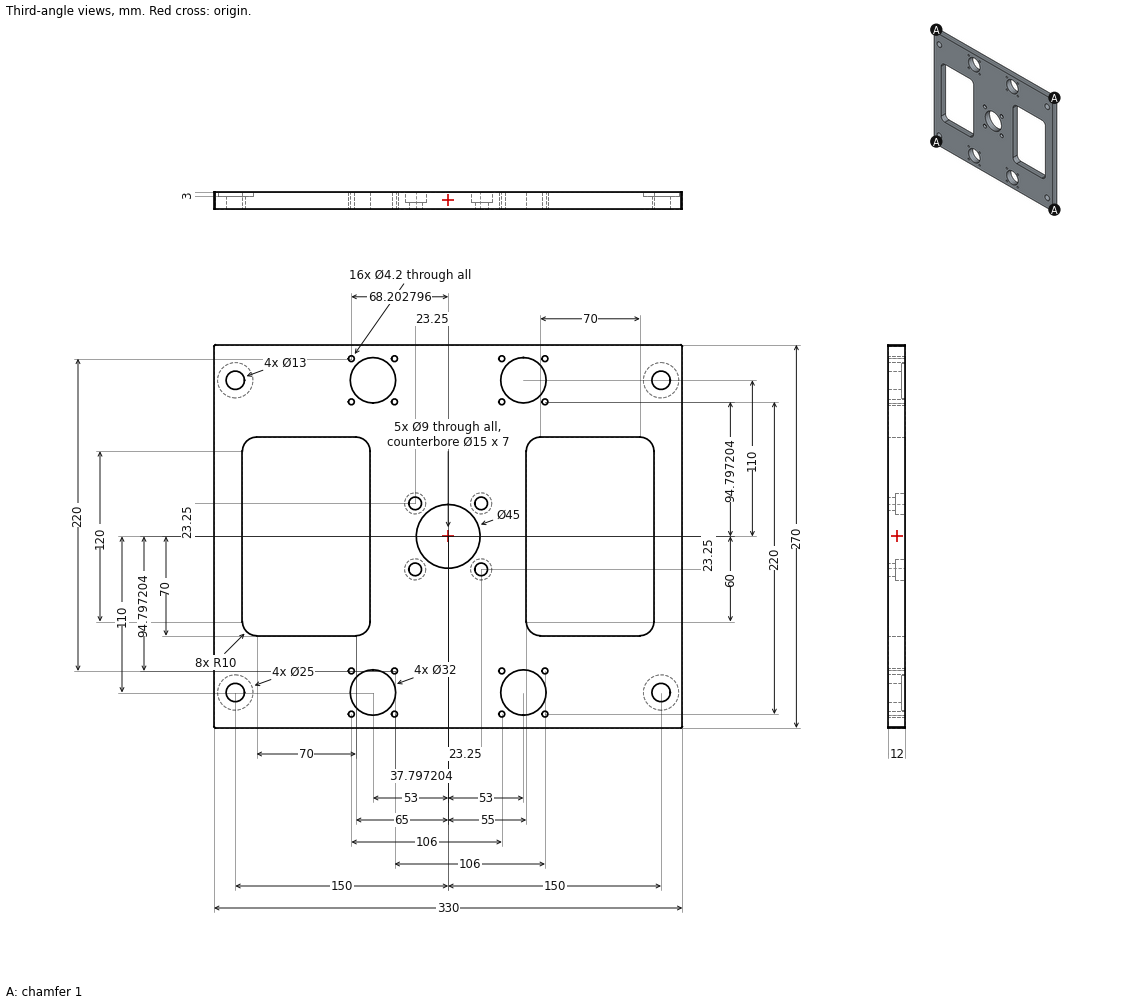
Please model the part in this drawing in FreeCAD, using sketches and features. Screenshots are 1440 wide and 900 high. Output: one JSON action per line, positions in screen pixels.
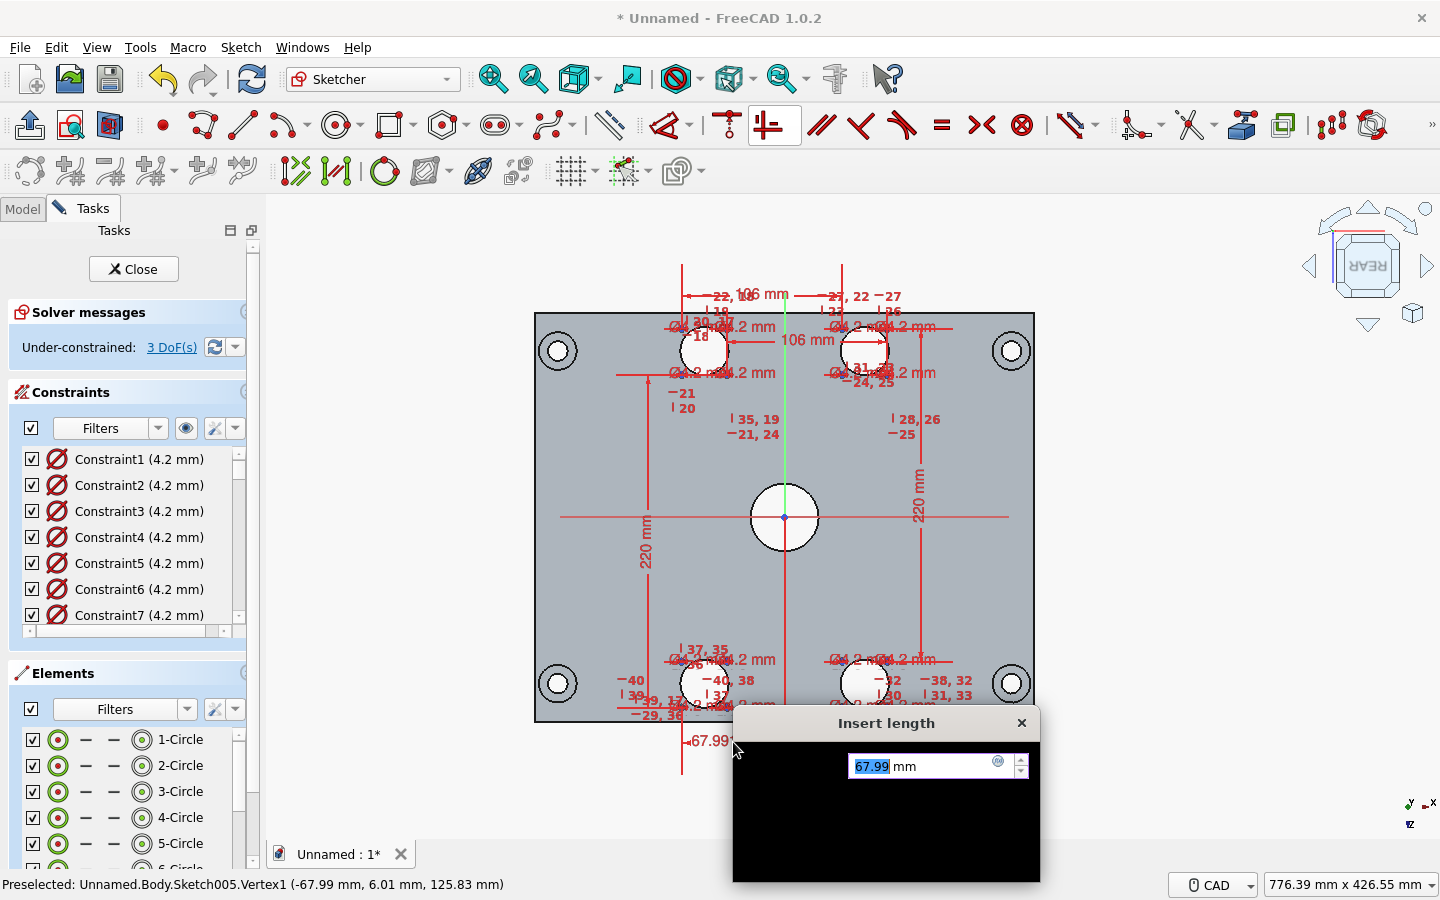
{"action": "type", "text": "68.202796"}
{"action": "key", "text": "Return"}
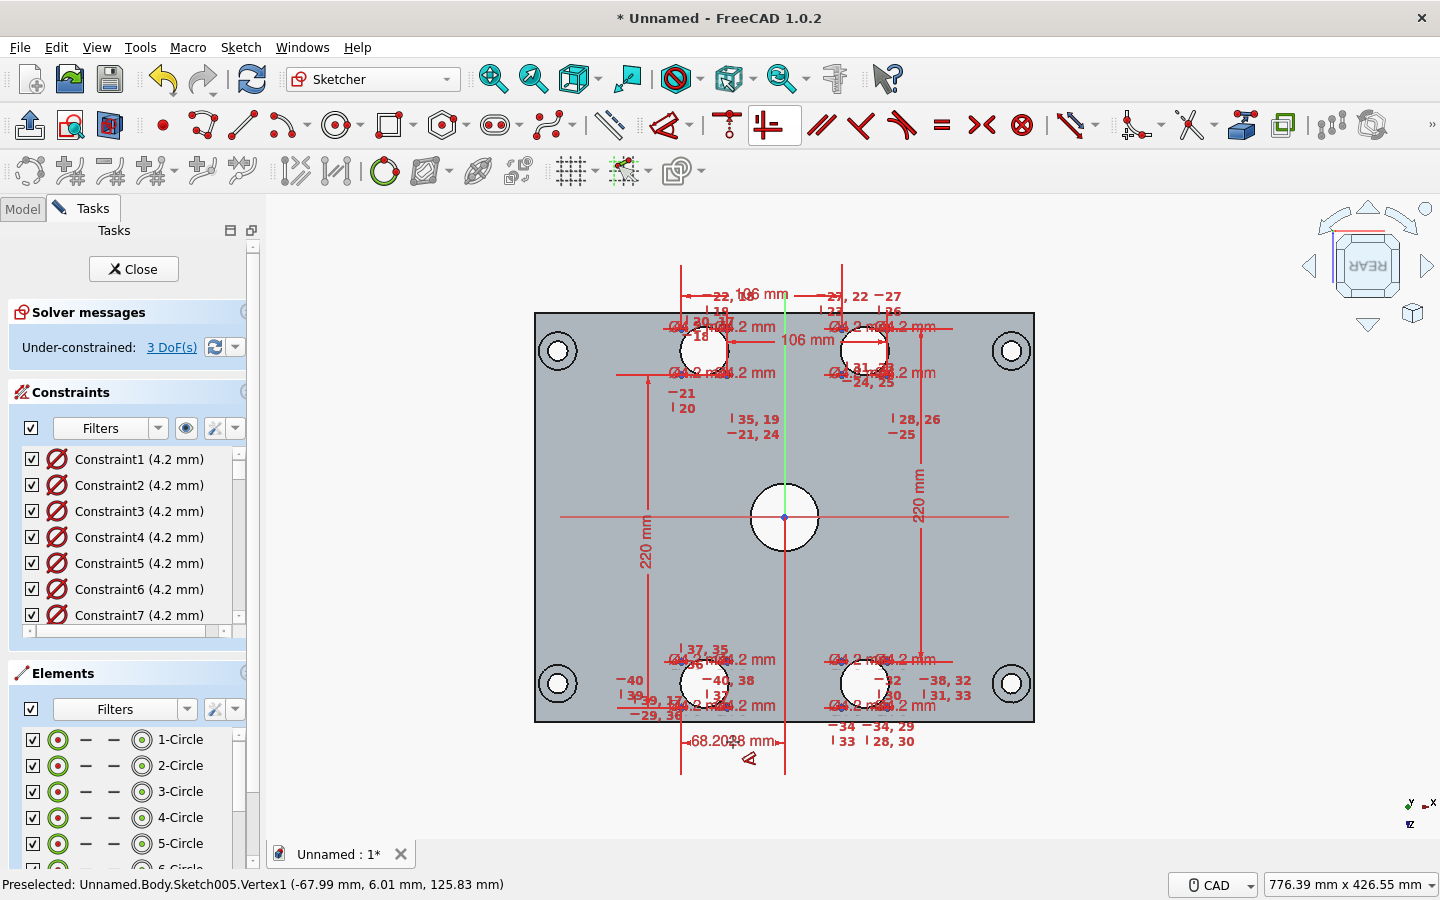
{"action": "left_click", "coordinate": [727, 329]}
{"action": "left_click", "coordinate": [756, 551]}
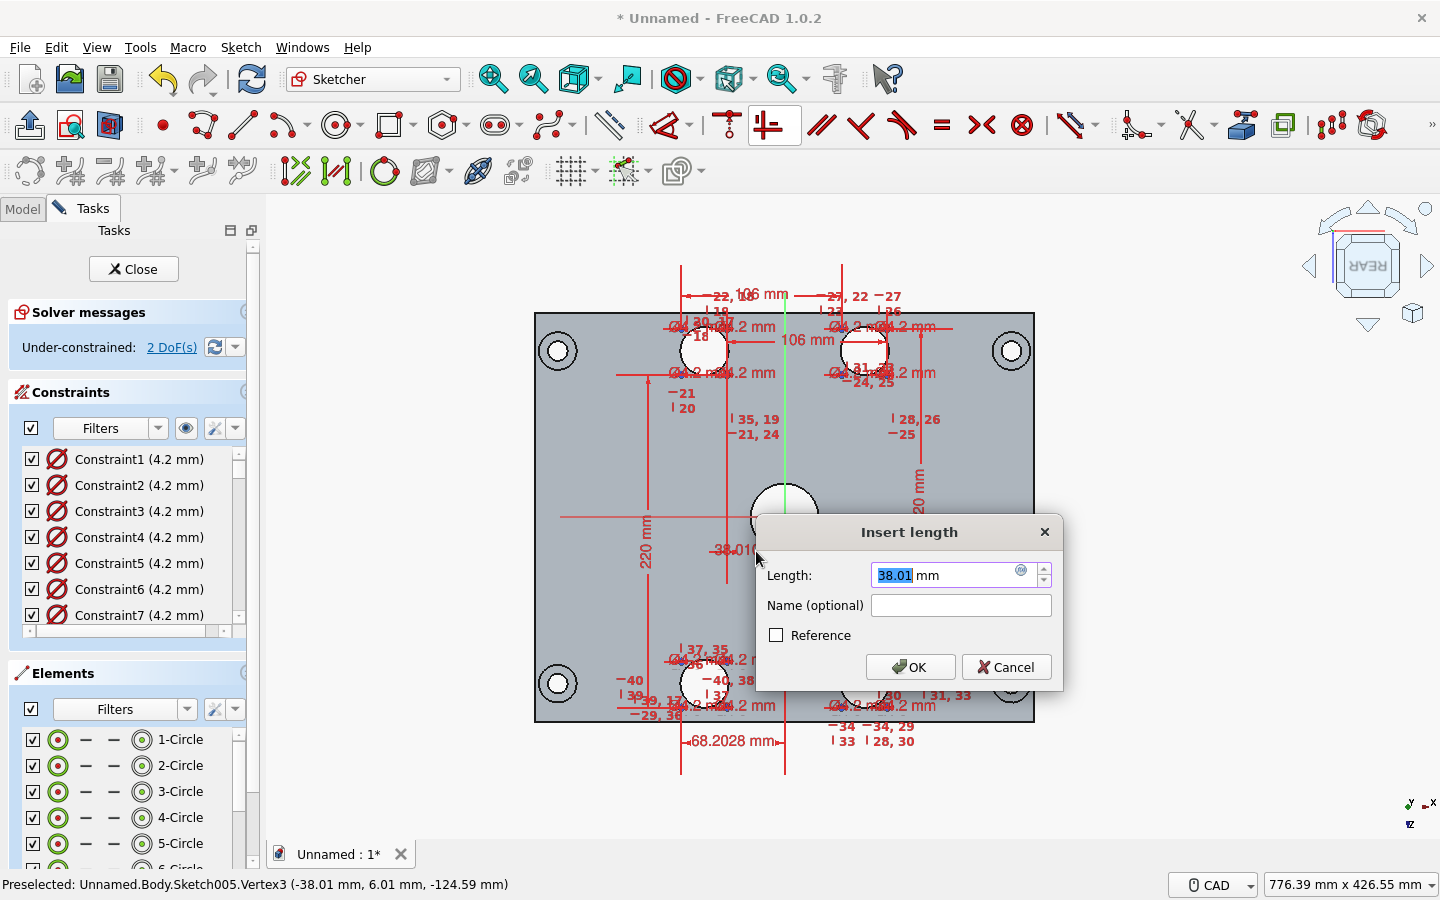
{"action": "type", "text": "37.797204"}
{"action": "key", "text": "Return"}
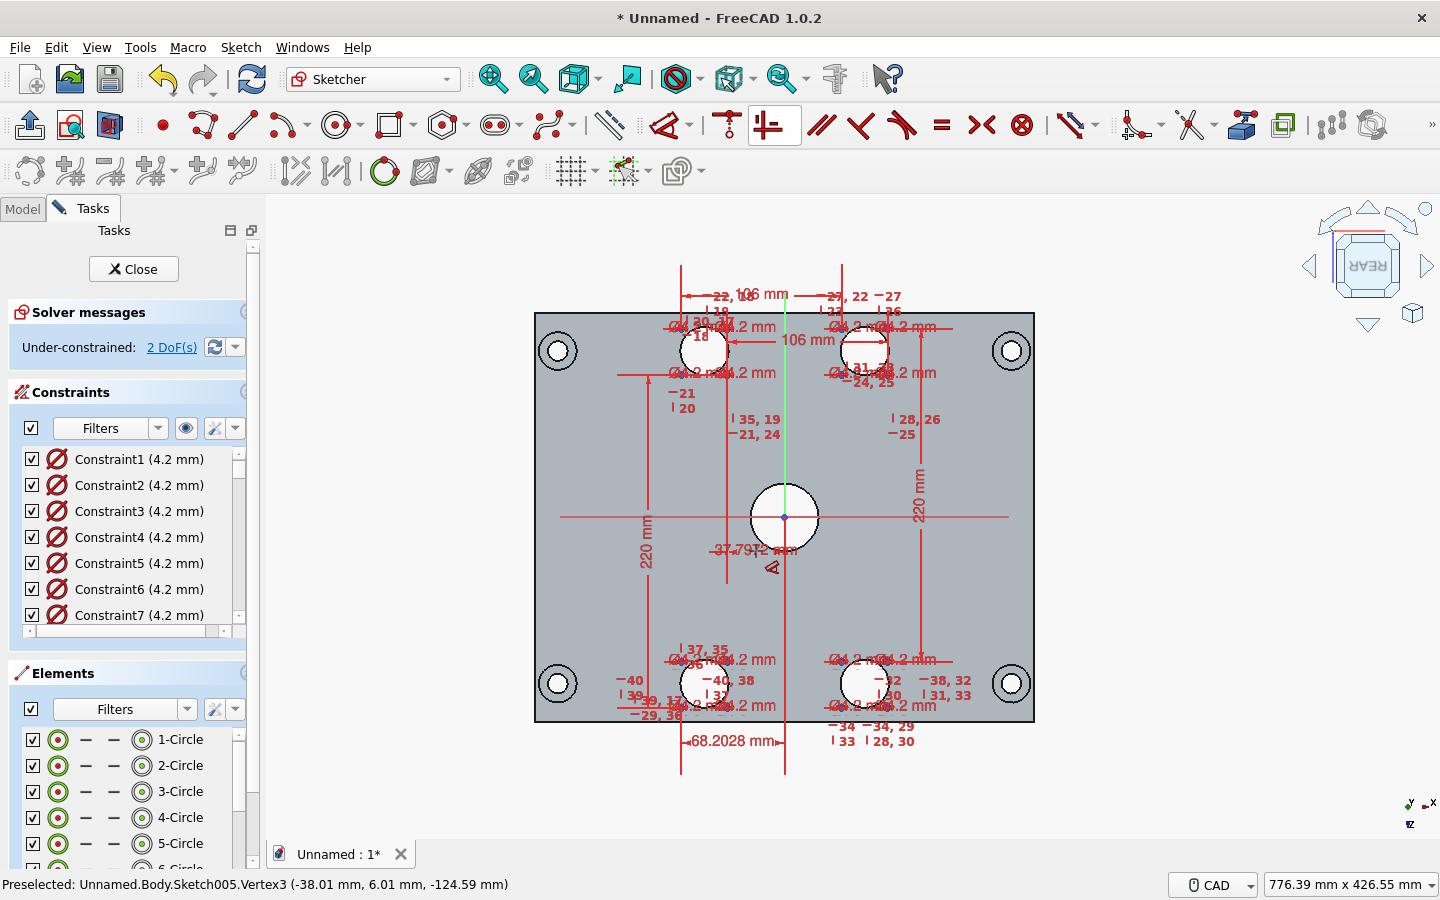
{"action": "left_click", "coordinate": [727, 375]}
{"action": "left_click", "coordinate": [693, 446]}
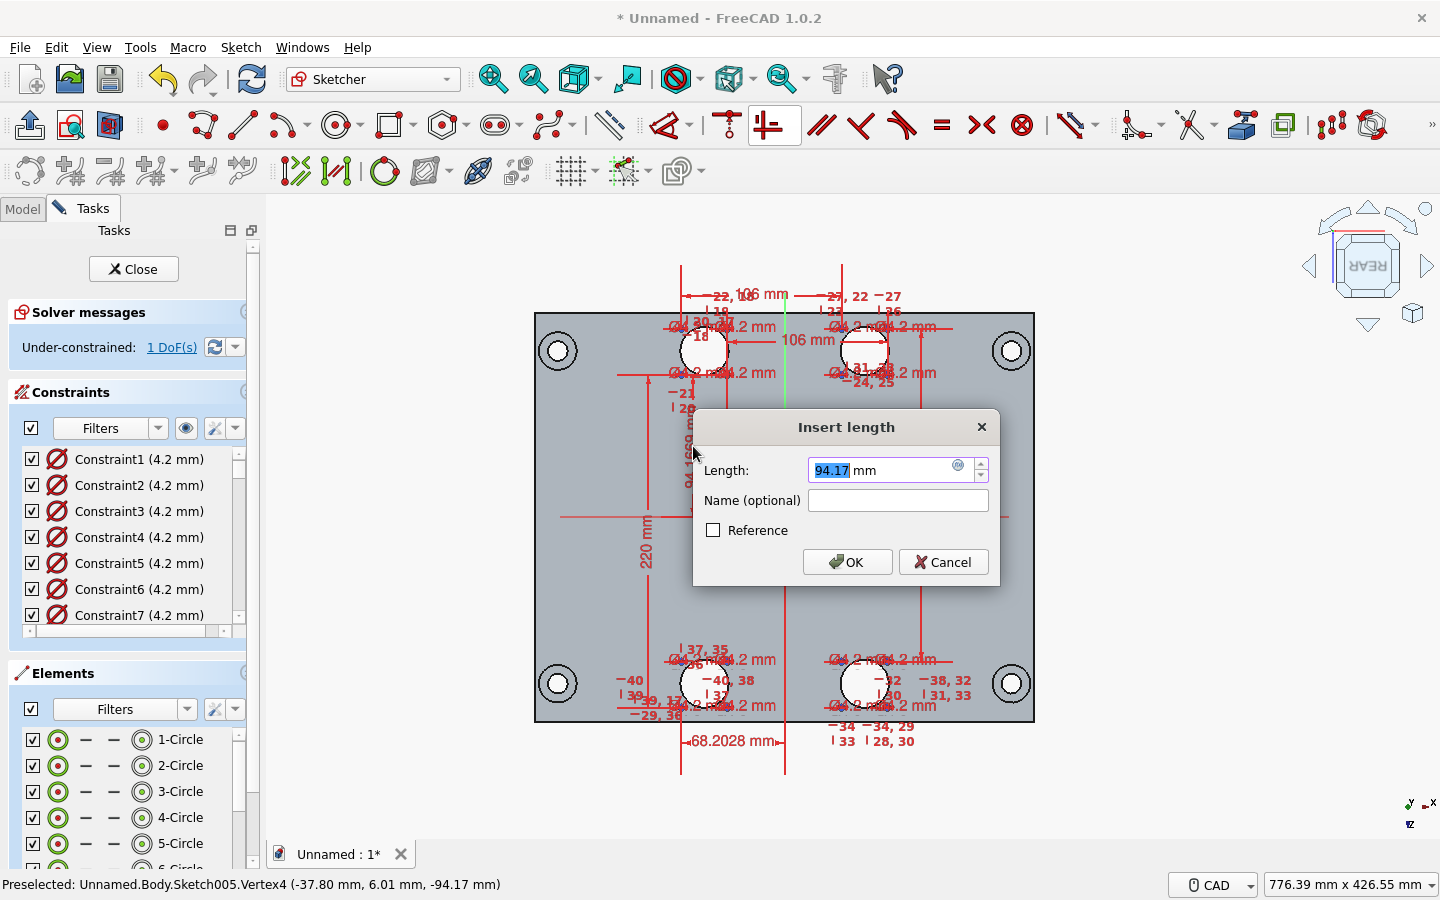
{"action": "type", "text": "94.797204"}
{"action": "key", "text": "Return"}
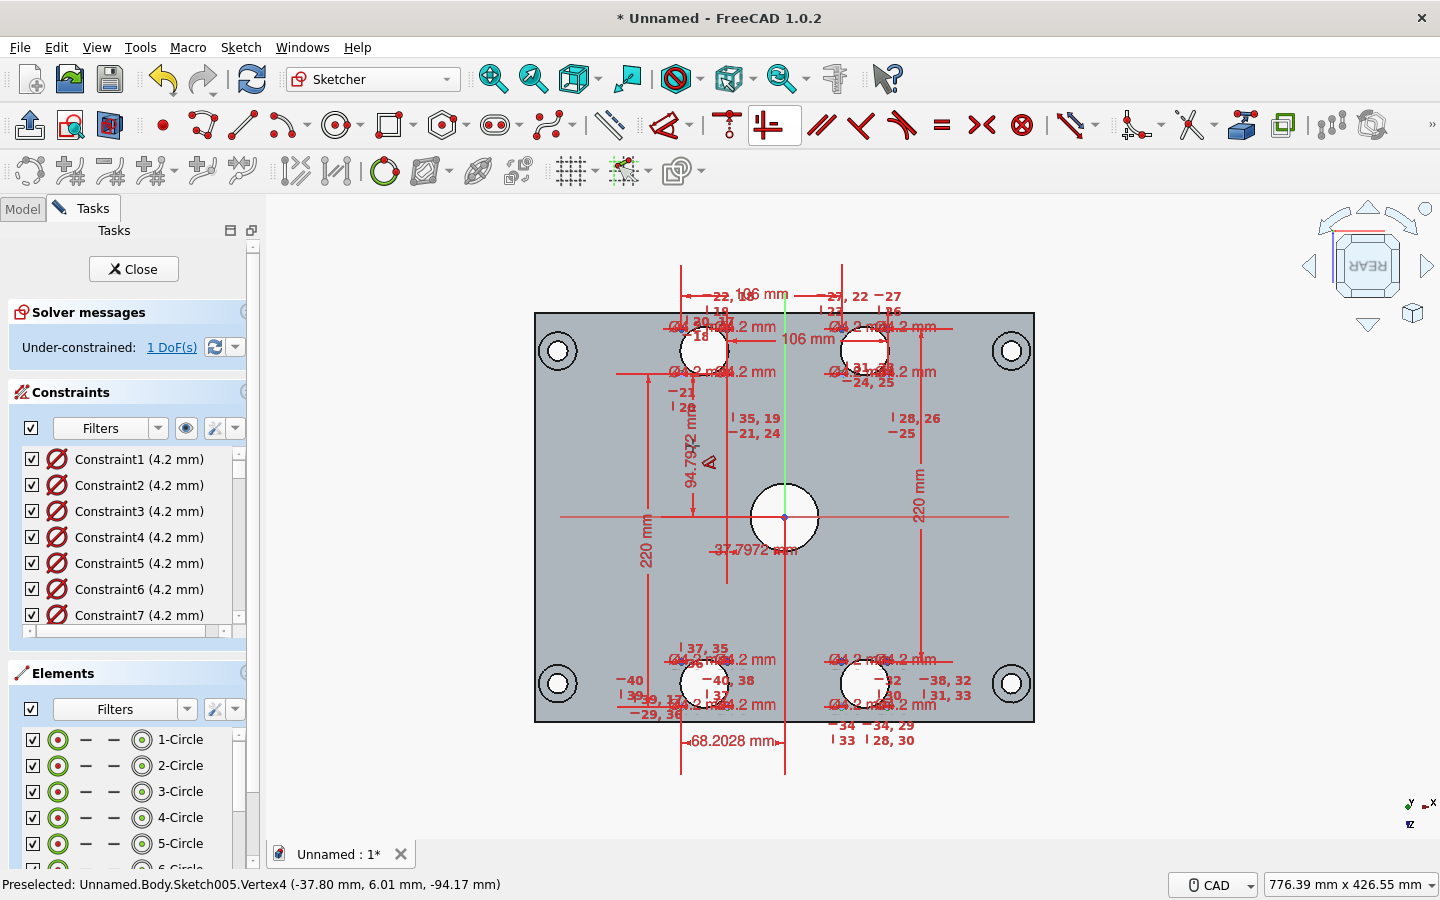
{"action": "left_click", "coordinate": [888, 662]}
{"action": "left_click", "coordinate": [922, 590]}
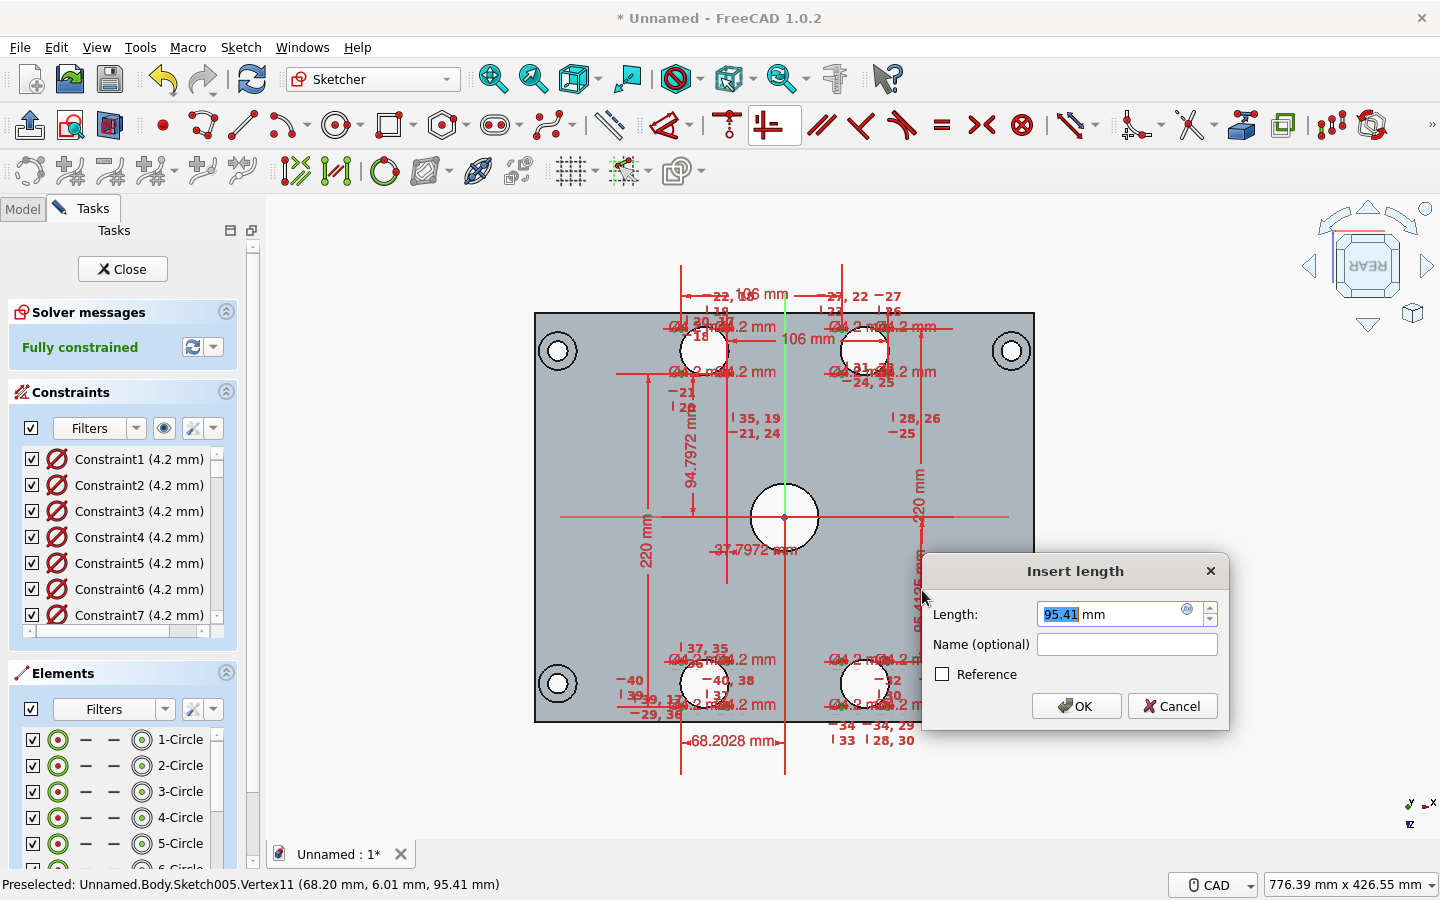
{"action": "type", "text": "94.797204"}
{"action": "key", "text": "Return"}
{"action": "key", "text": "Escape"}